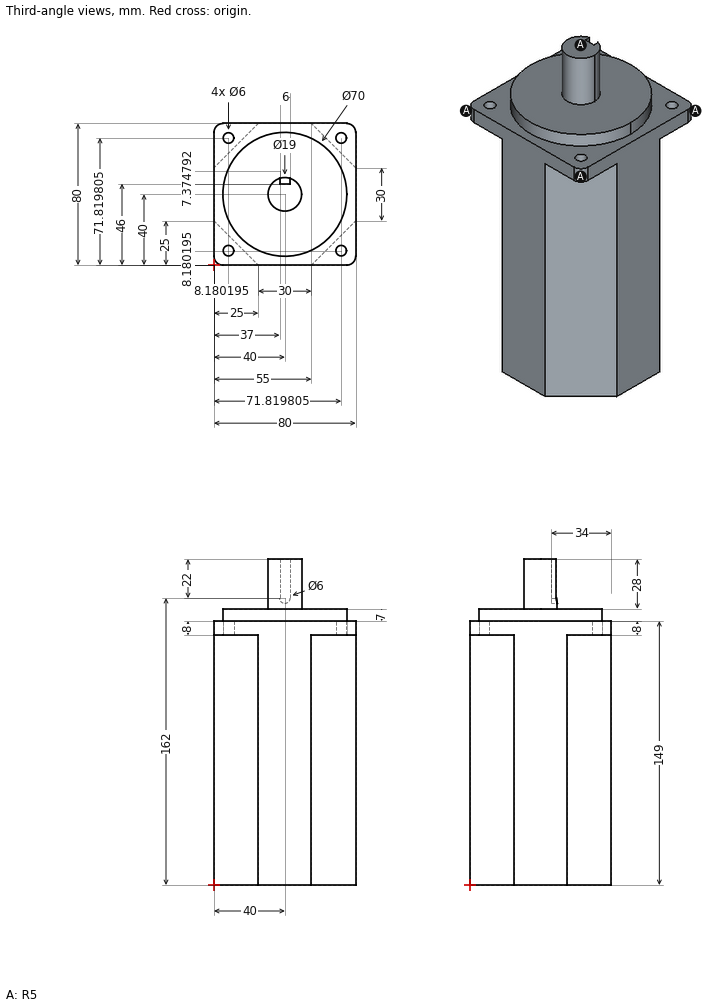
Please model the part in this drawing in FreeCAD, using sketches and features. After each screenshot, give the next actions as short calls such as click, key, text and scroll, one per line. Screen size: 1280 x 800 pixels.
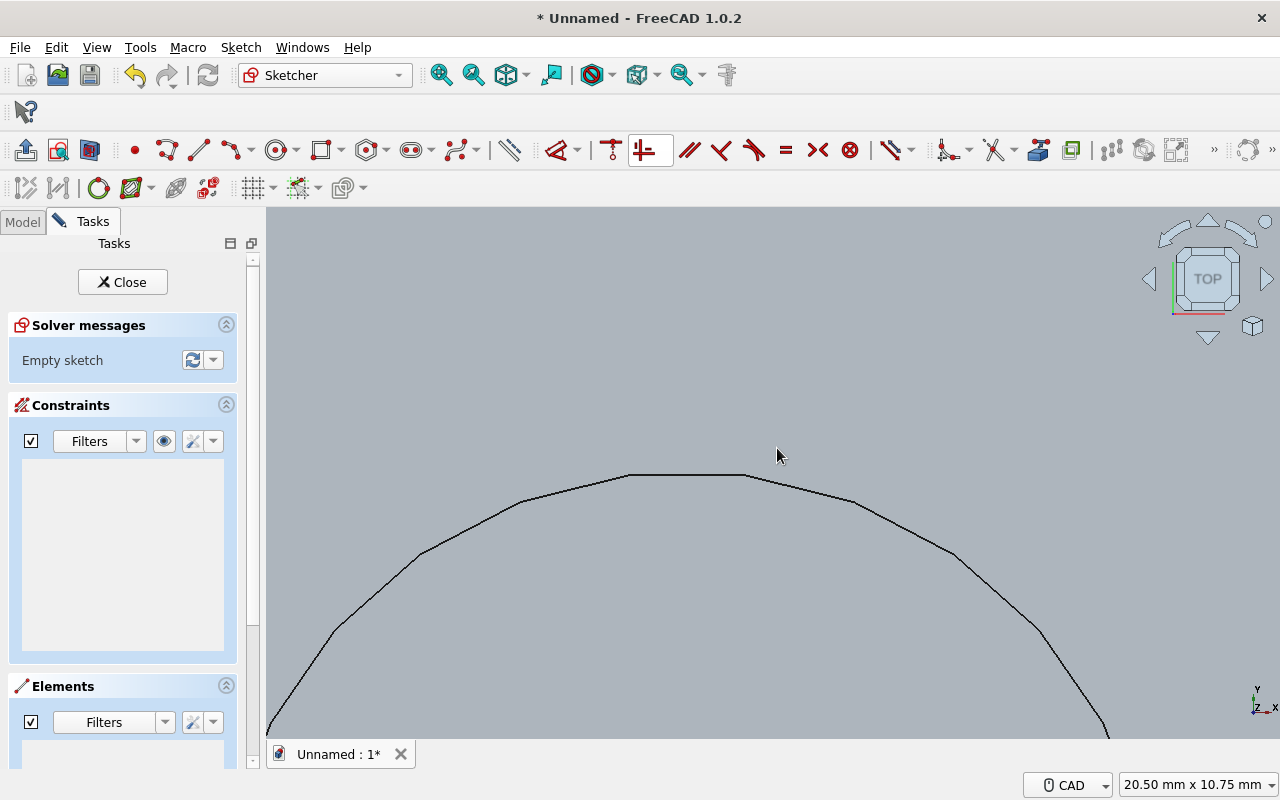
click(322, 150)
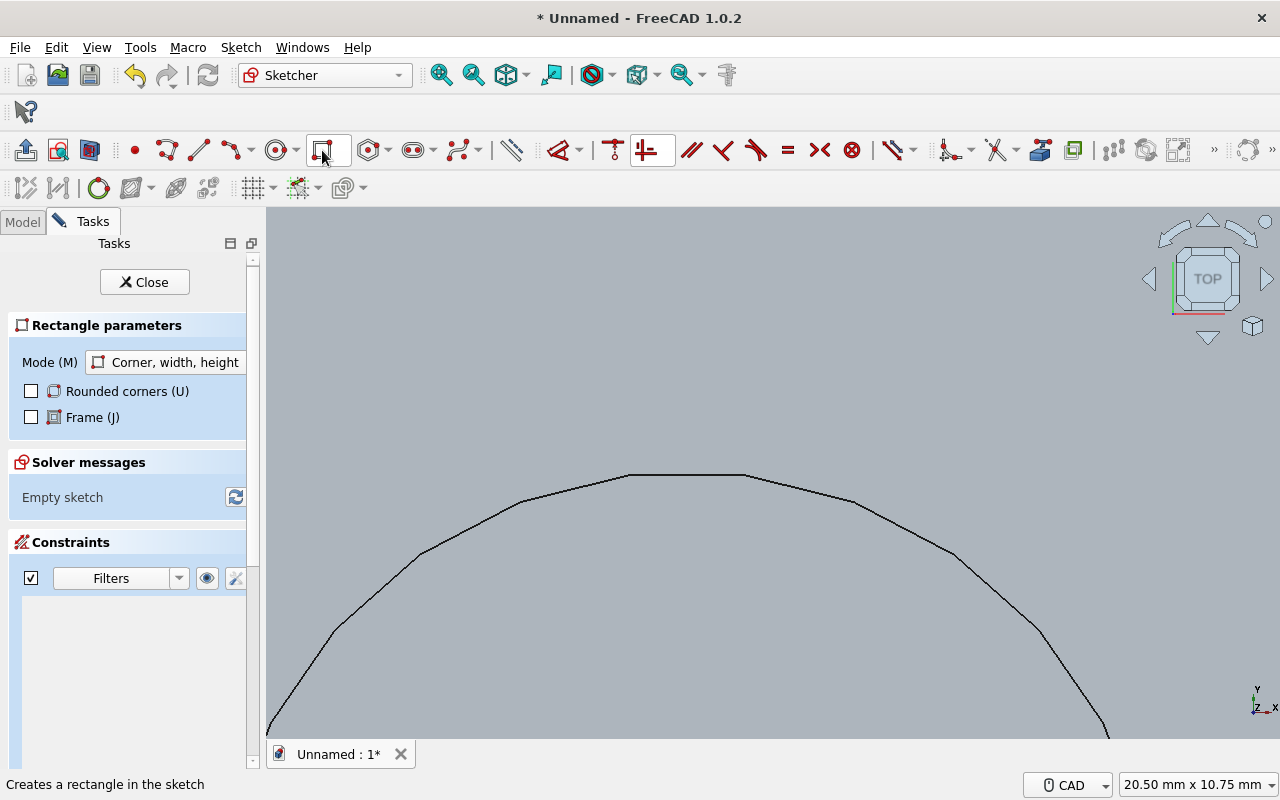
click(539, 280)
click(835, 645)
key(Escape)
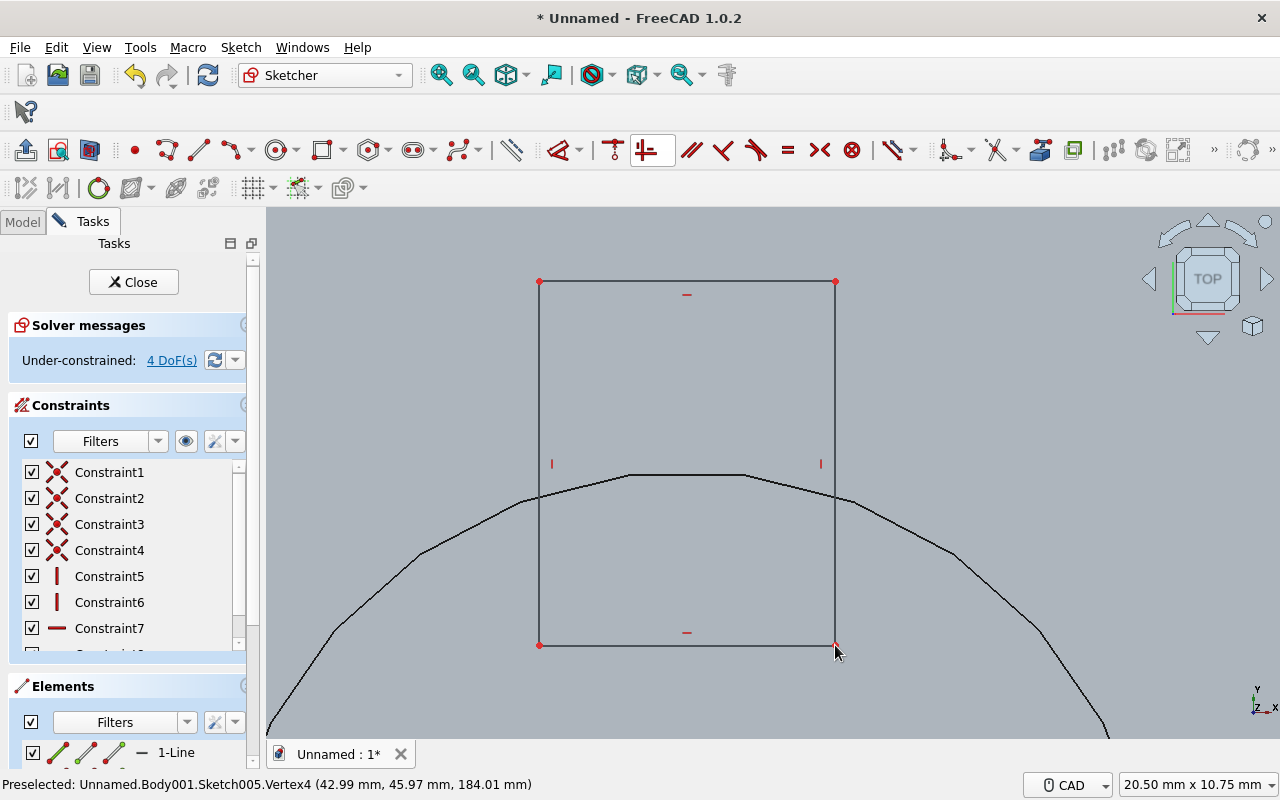
key(d)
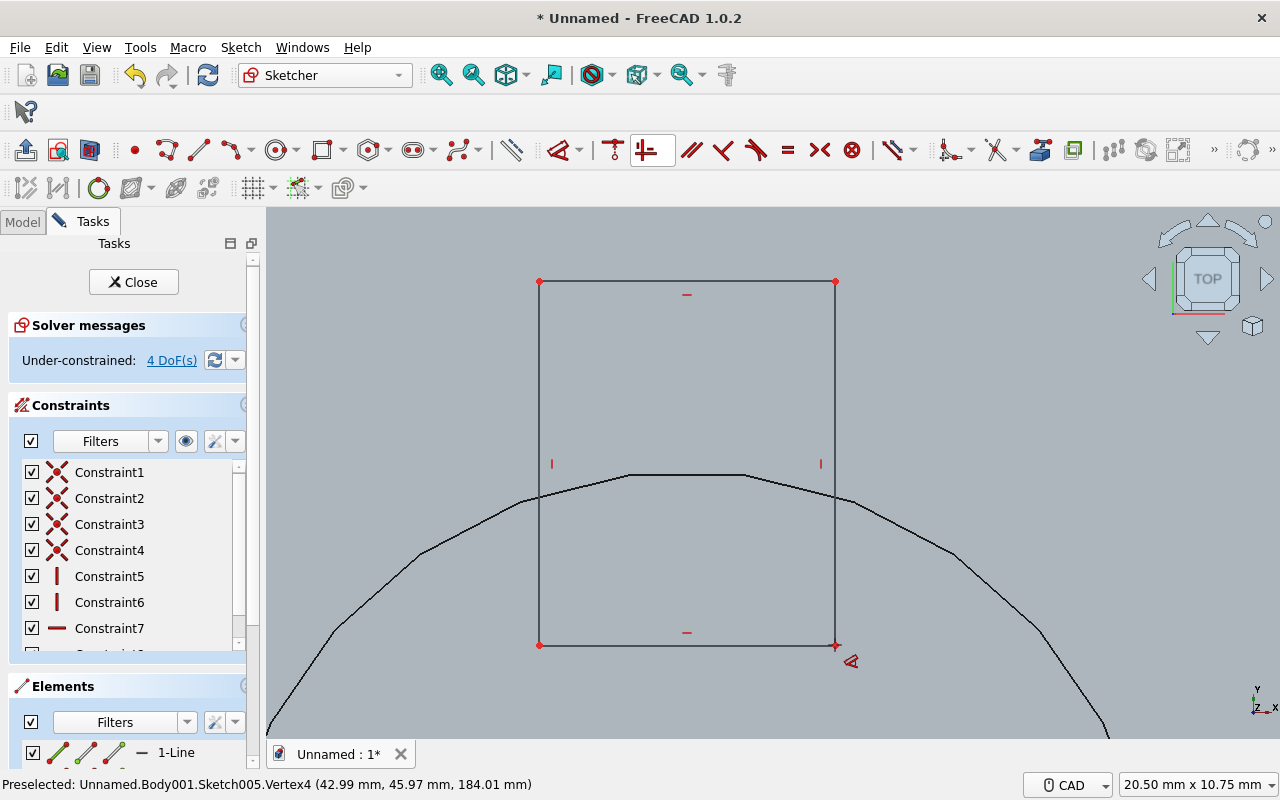
click(628, 646)
click(687, 680)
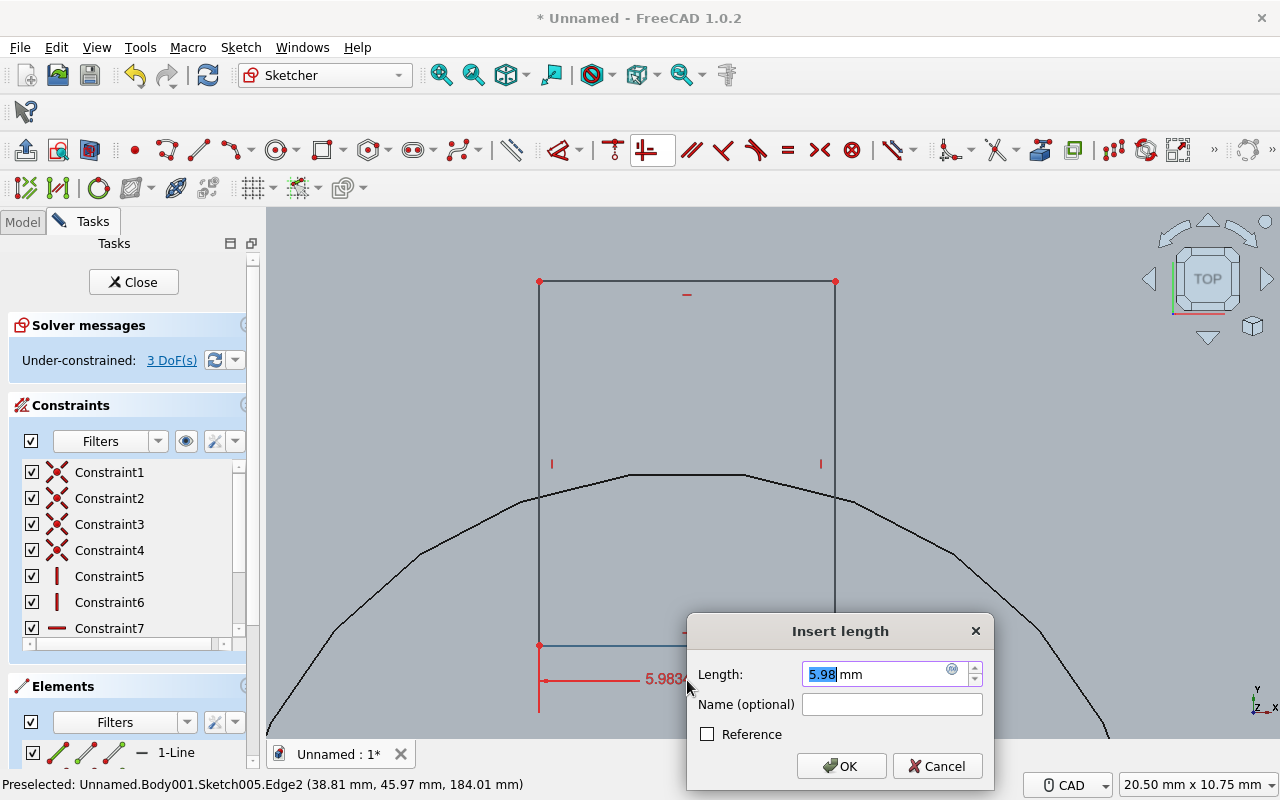
text(6)
key(Return)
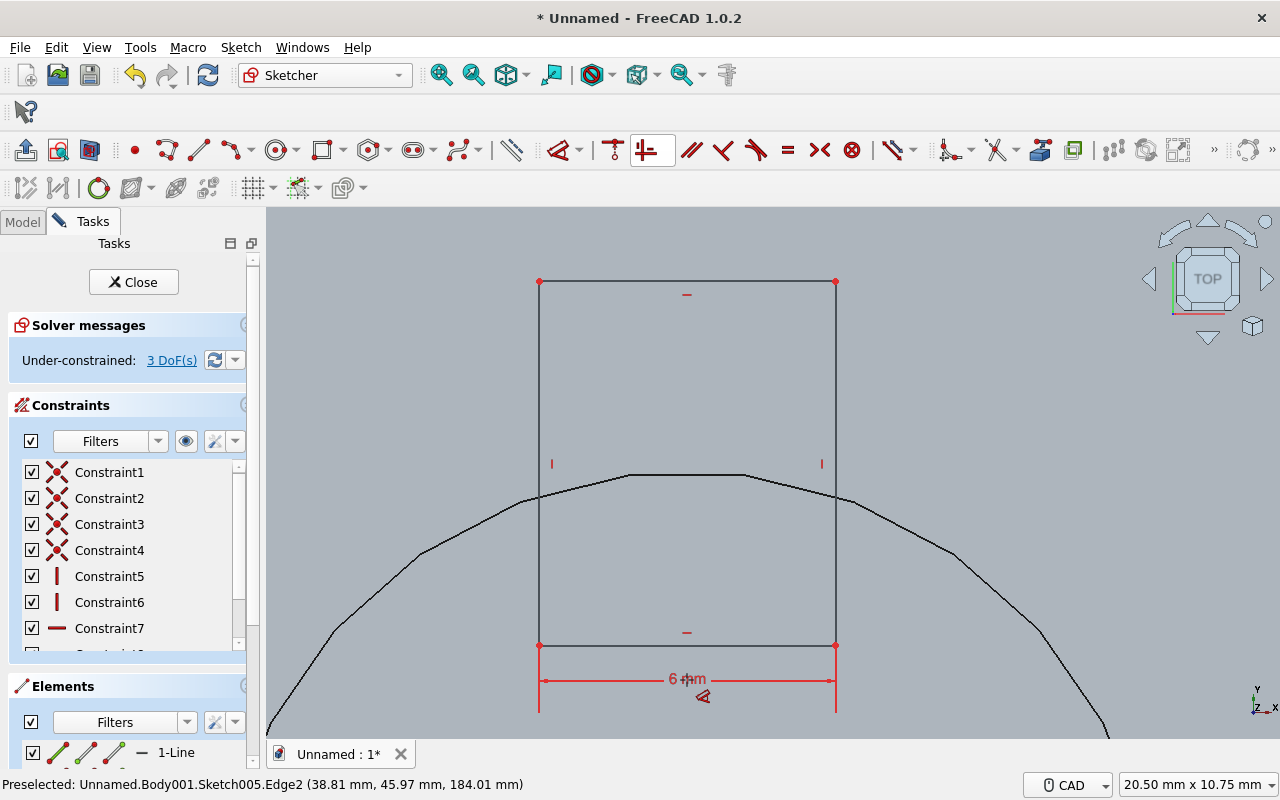
click(539, 281)
click(416, 247)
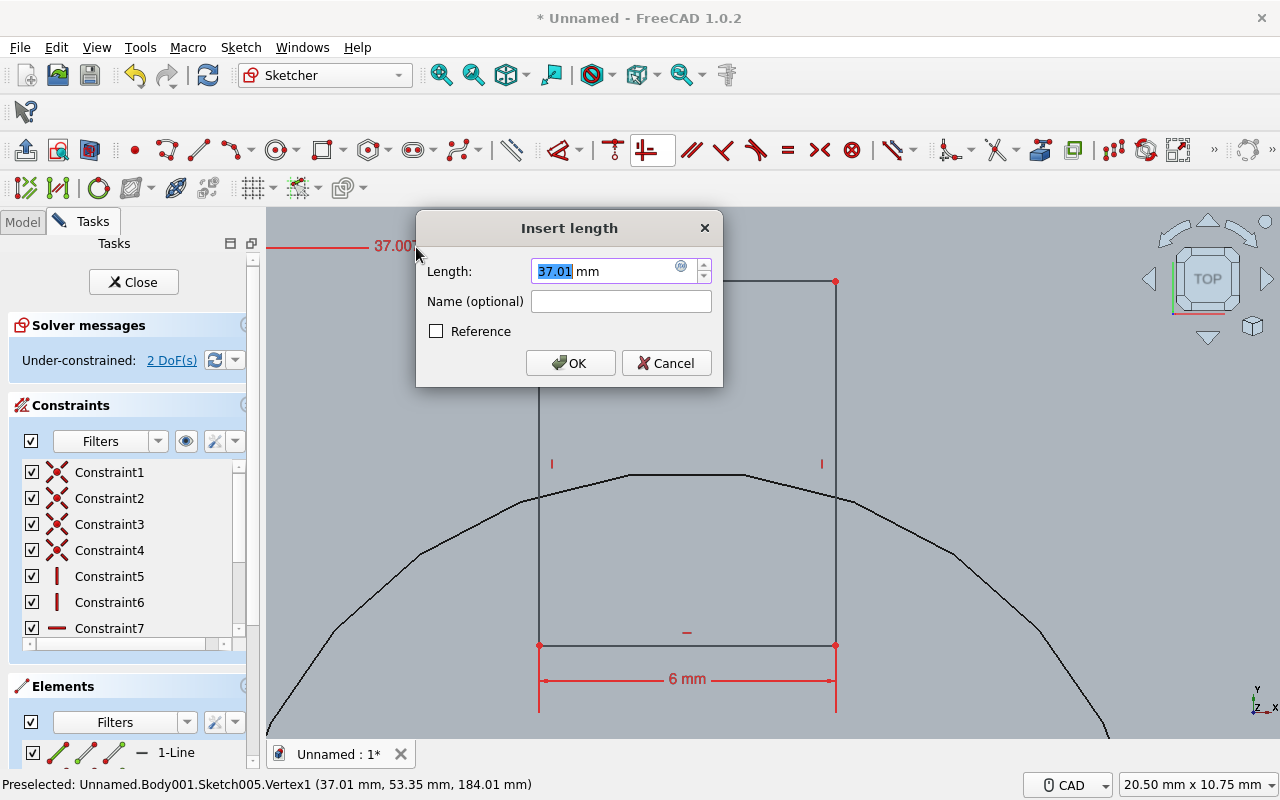
text(37)
key(Return)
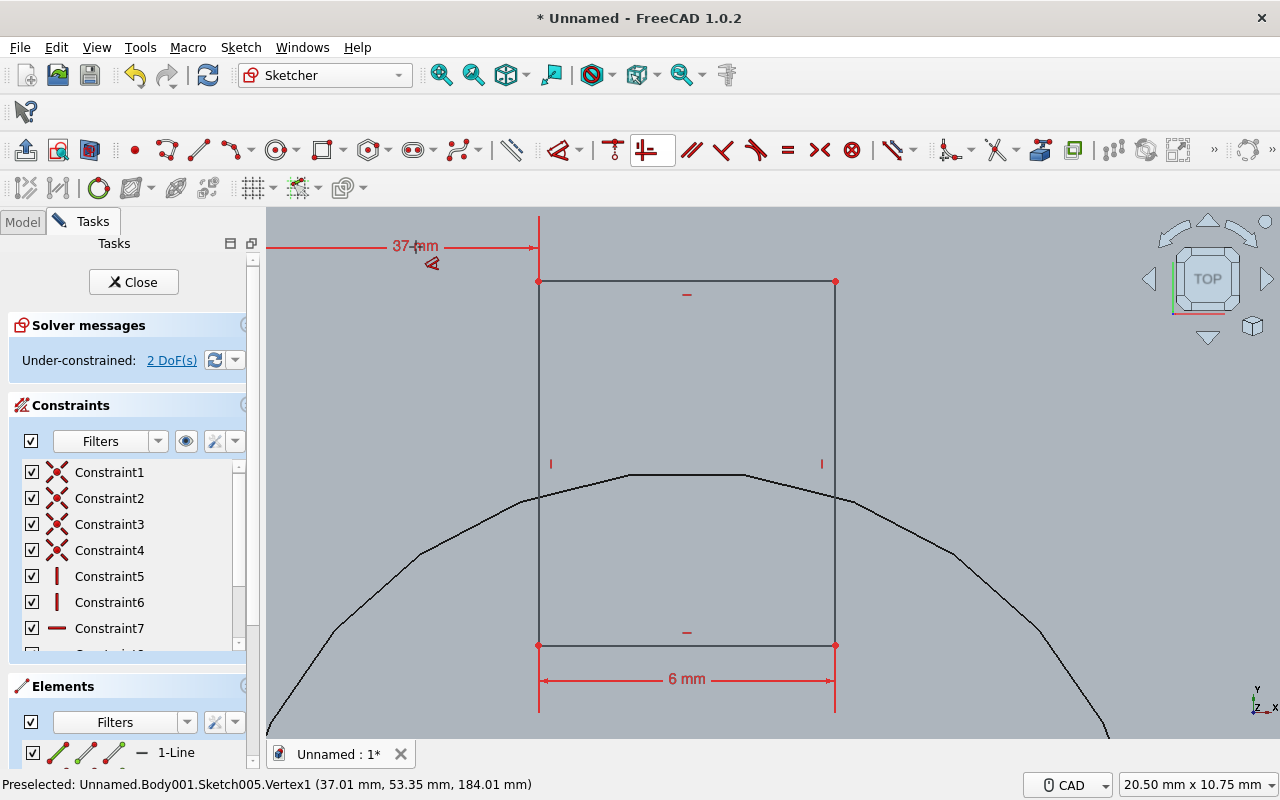
click(539, 646)
click(573, 678)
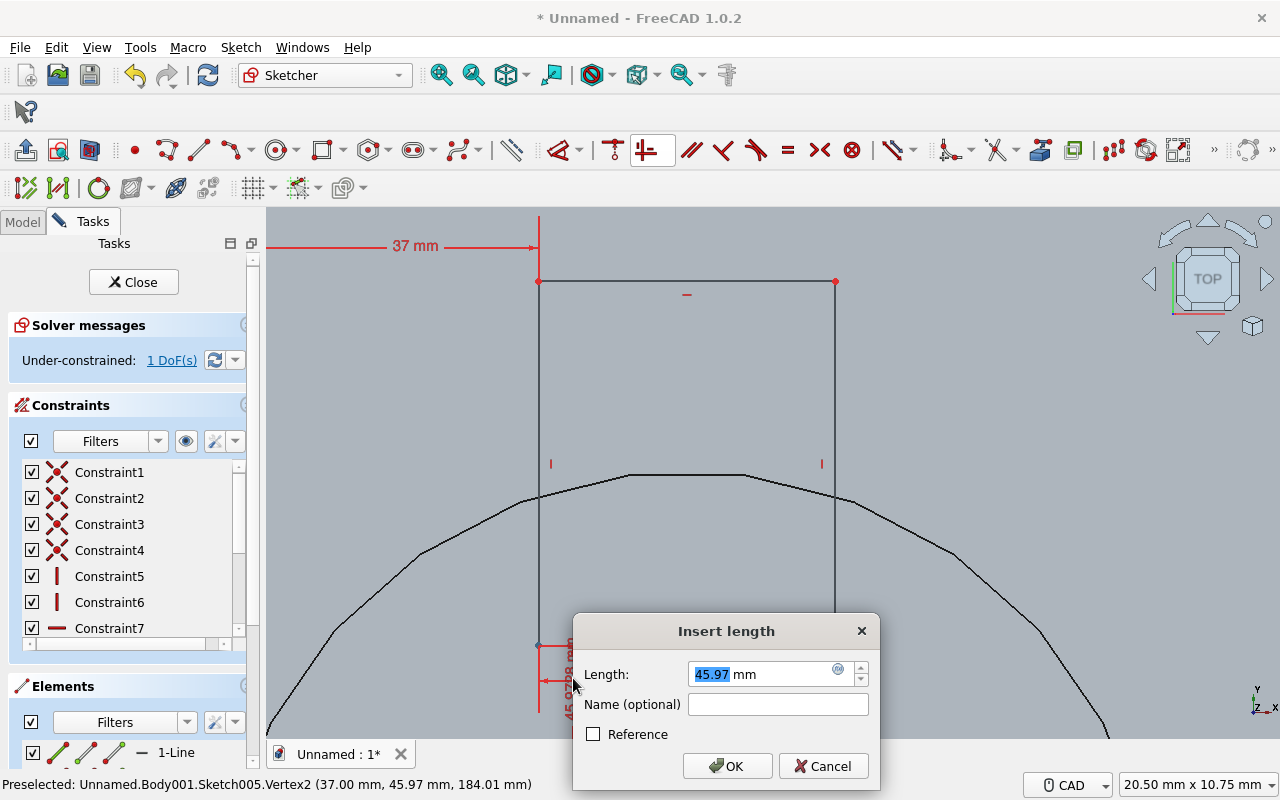
text(46)
key(Return)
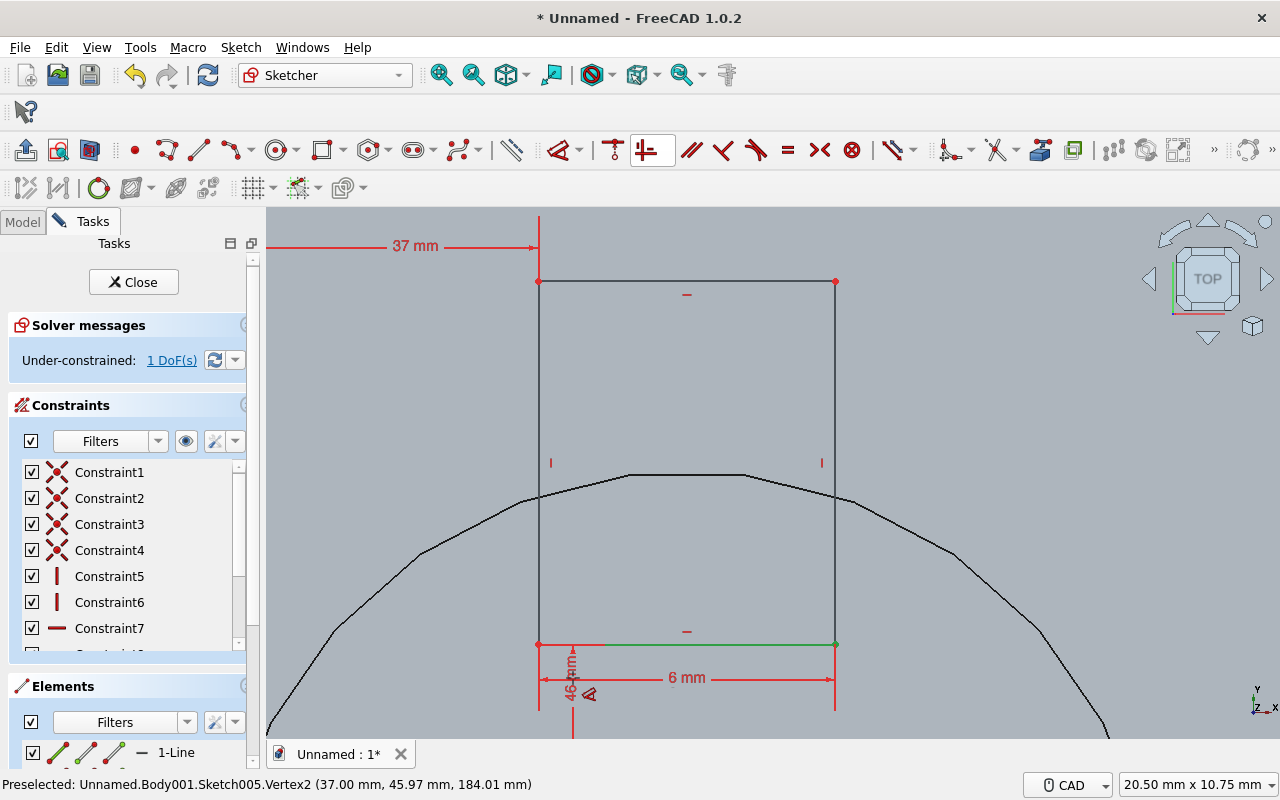
click(539, 390)
click(505, 463)